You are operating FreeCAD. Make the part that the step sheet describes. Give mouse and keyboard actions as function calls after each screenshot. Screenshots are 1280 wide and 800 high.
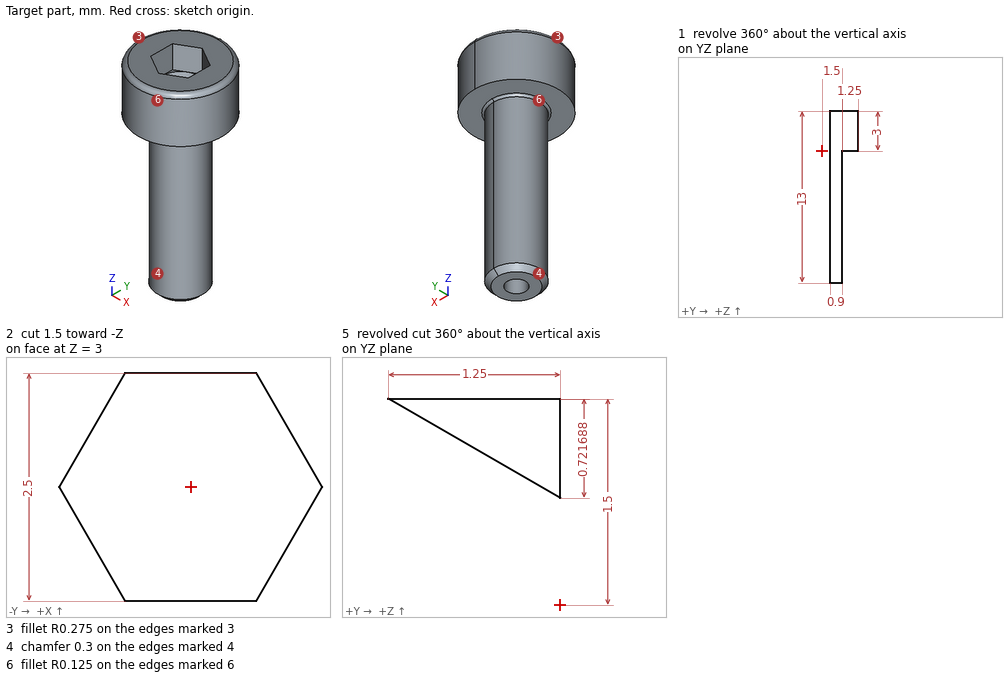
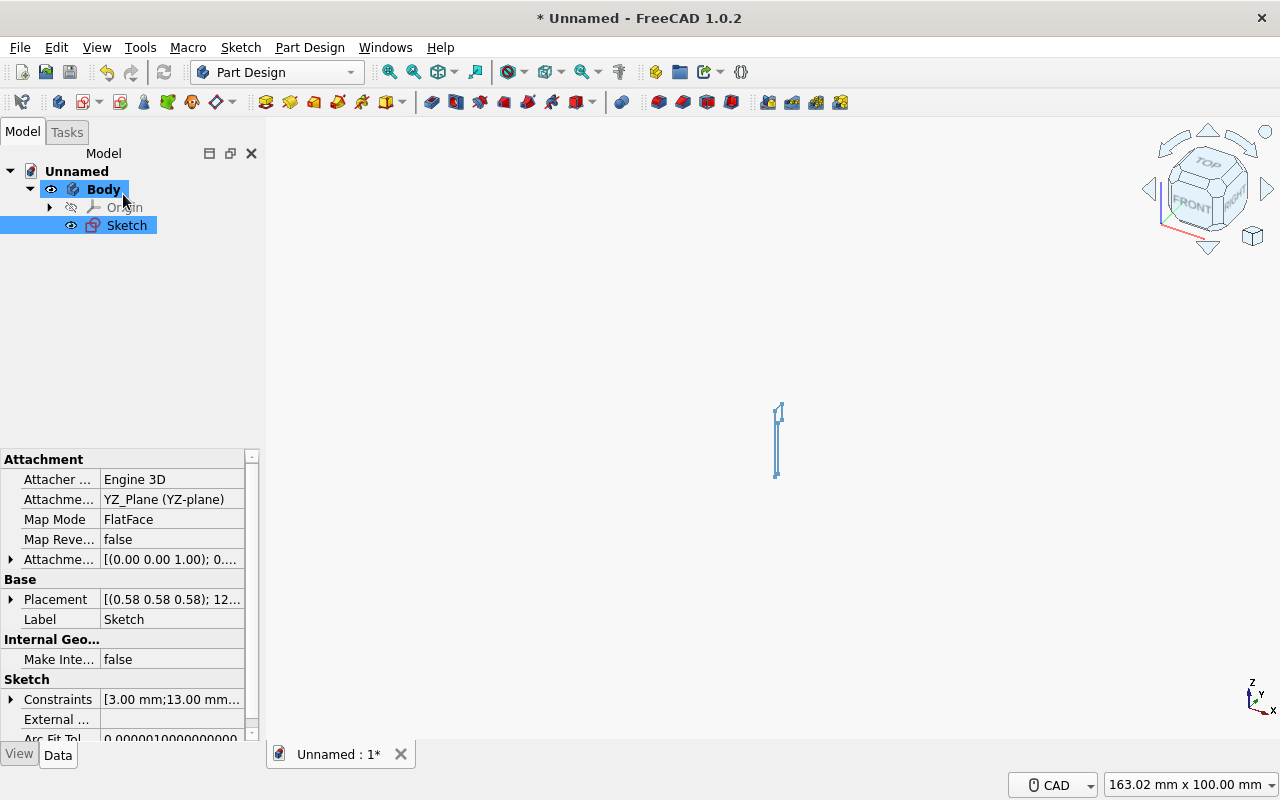
click(290, 102)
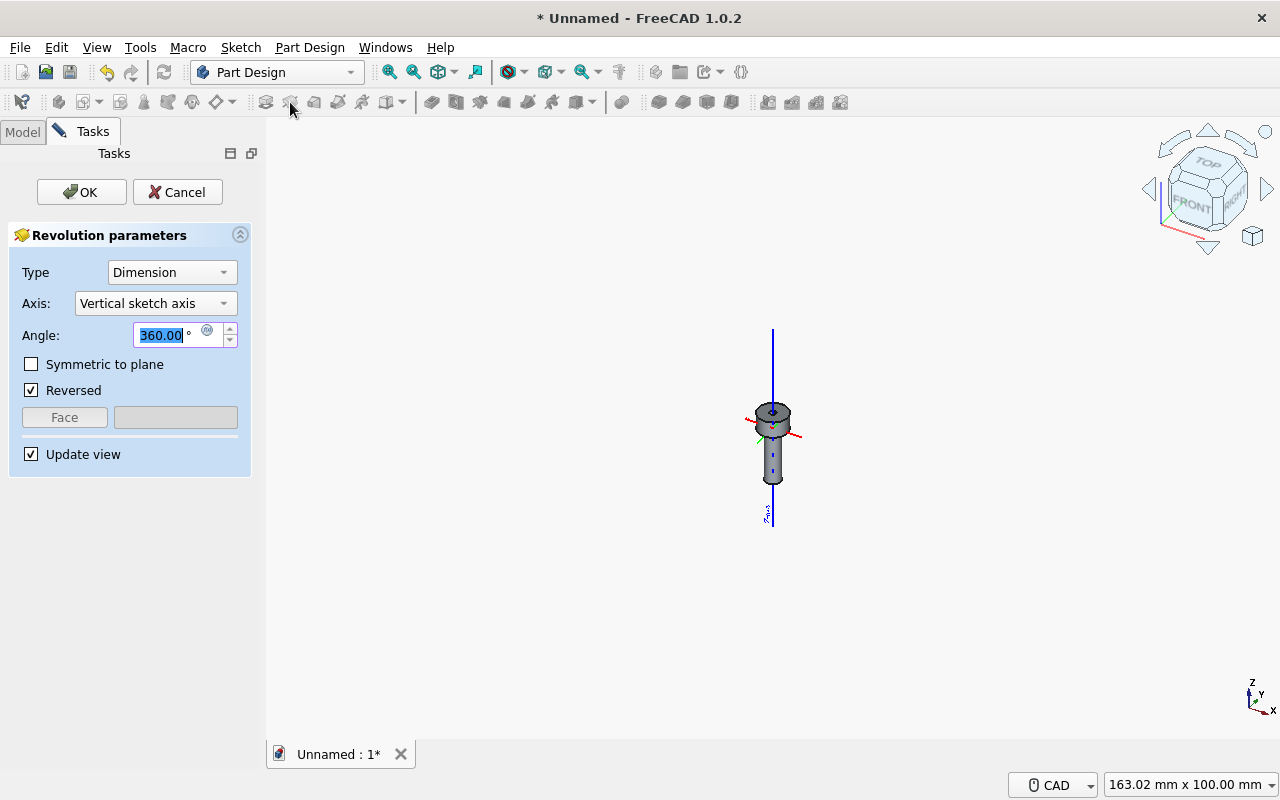
click(82, 192)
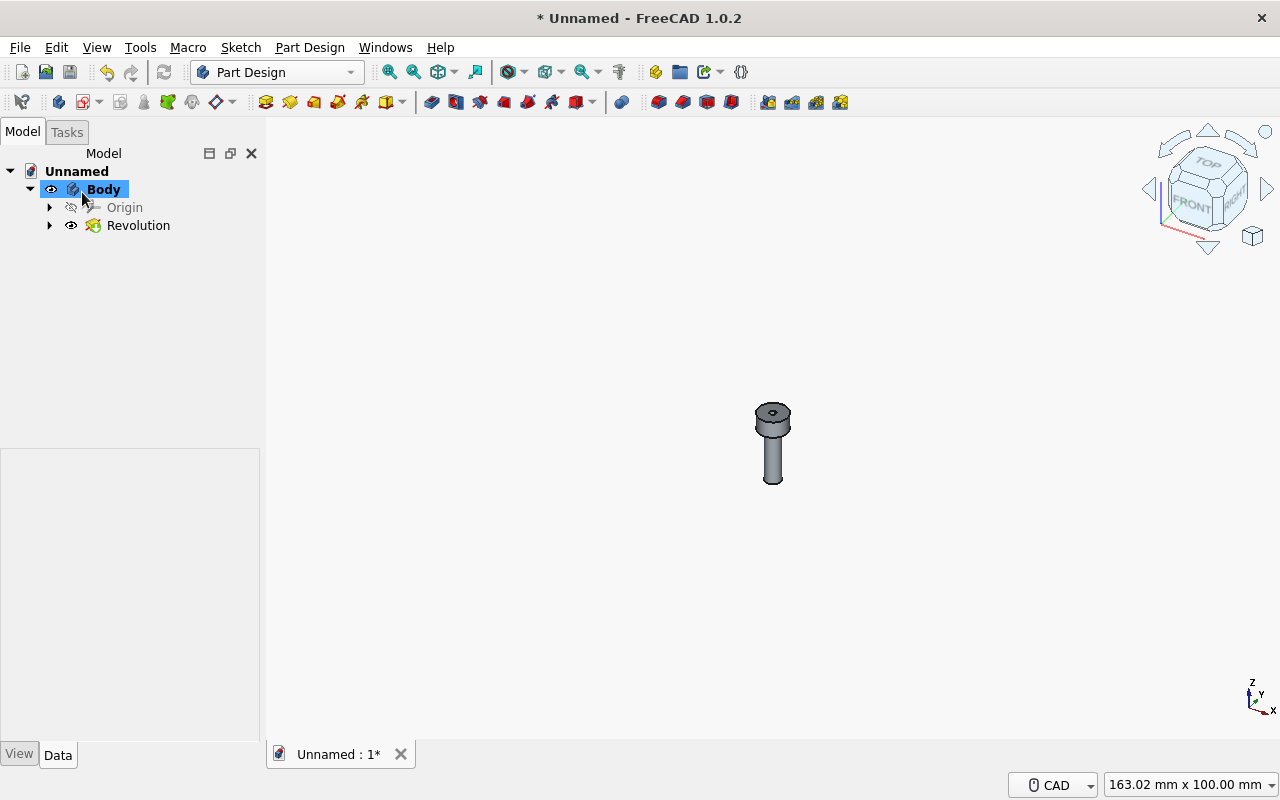
click(390, 72)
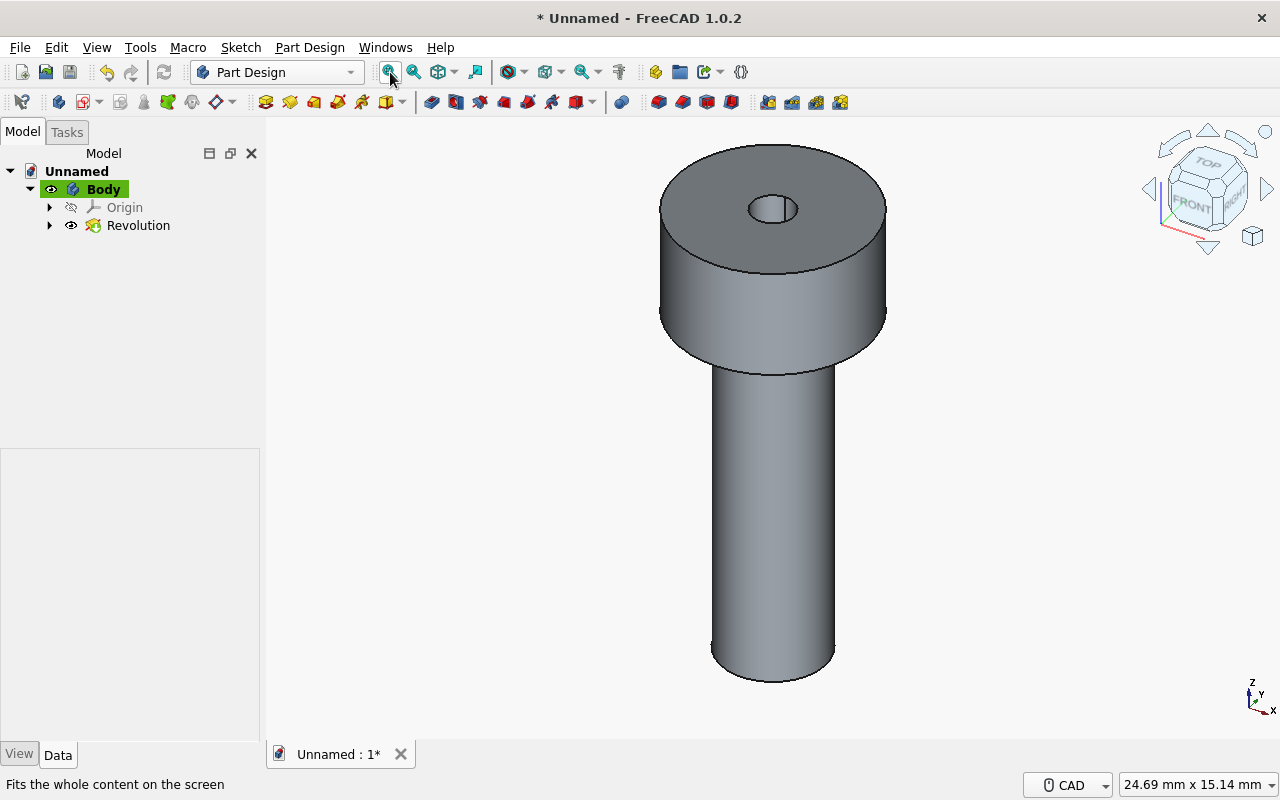
click(845, 211)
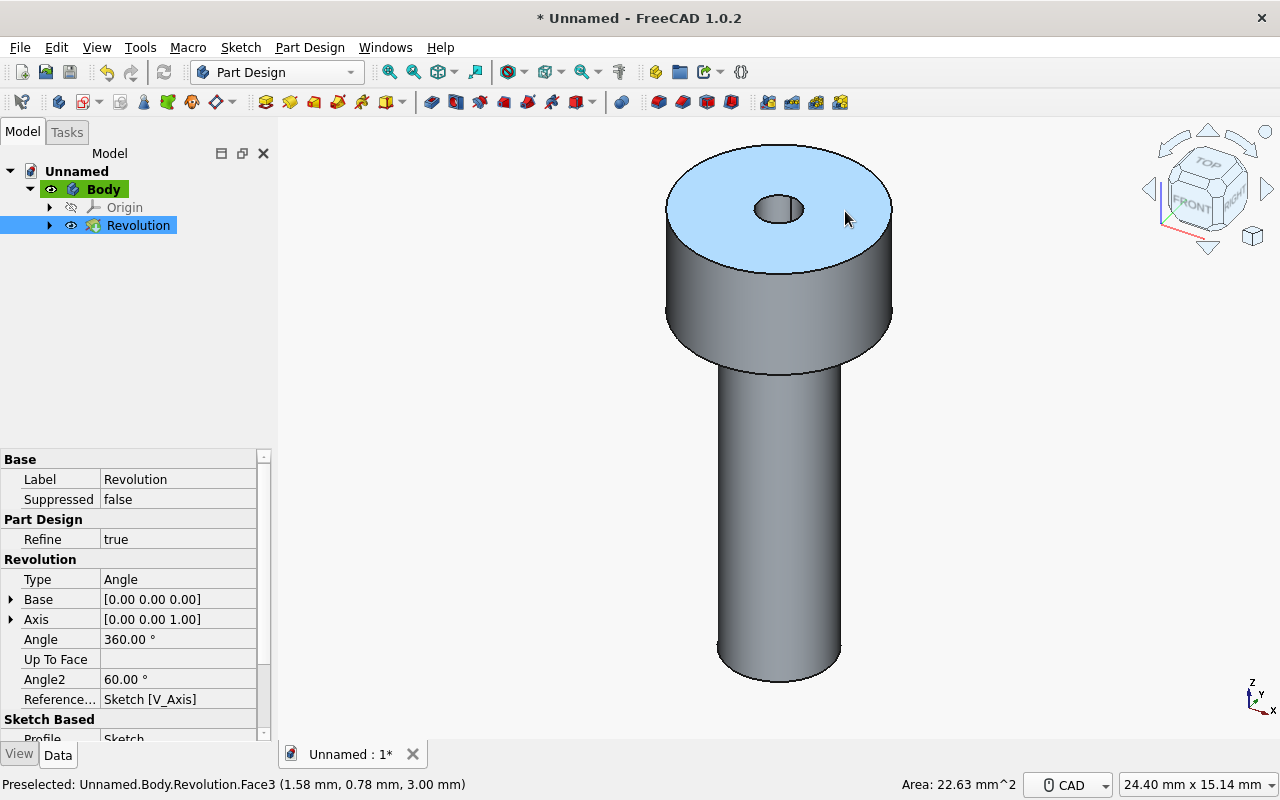
click(84, 102)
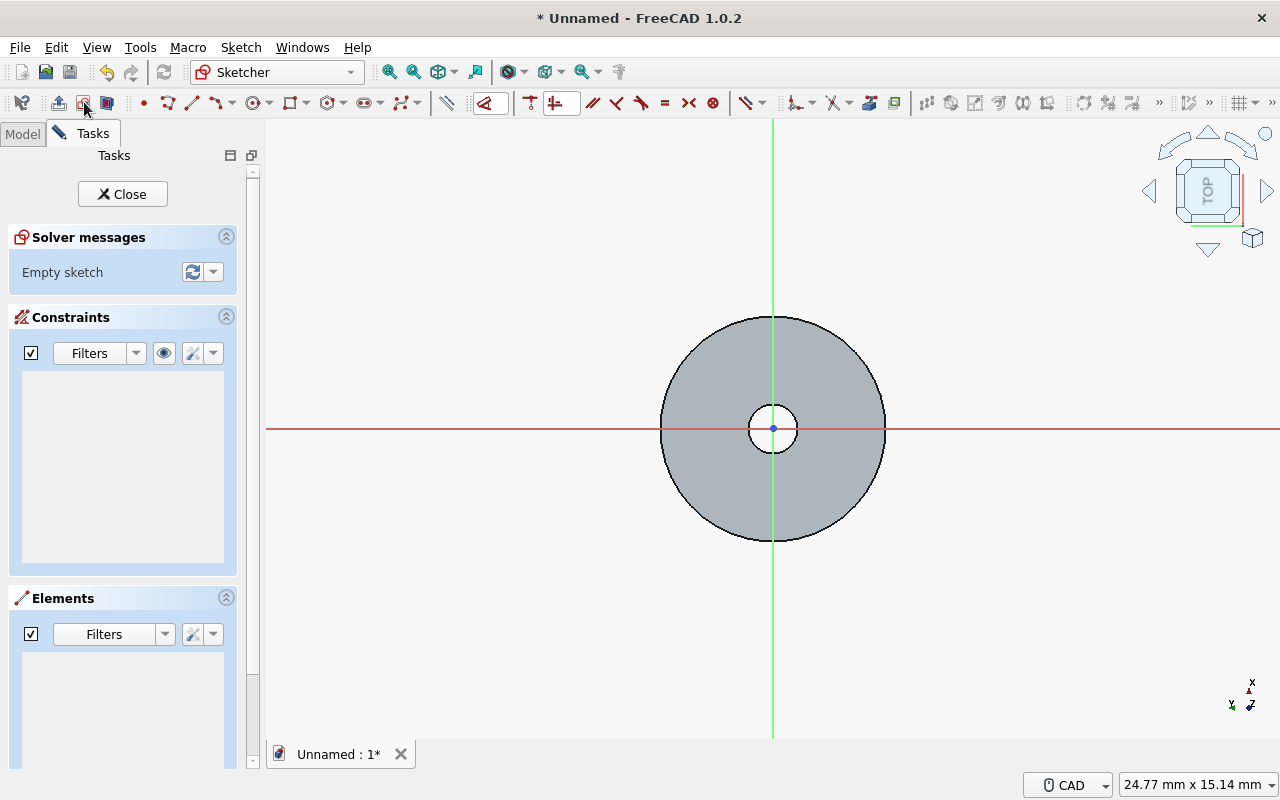
scroll(795, 429, up, 7)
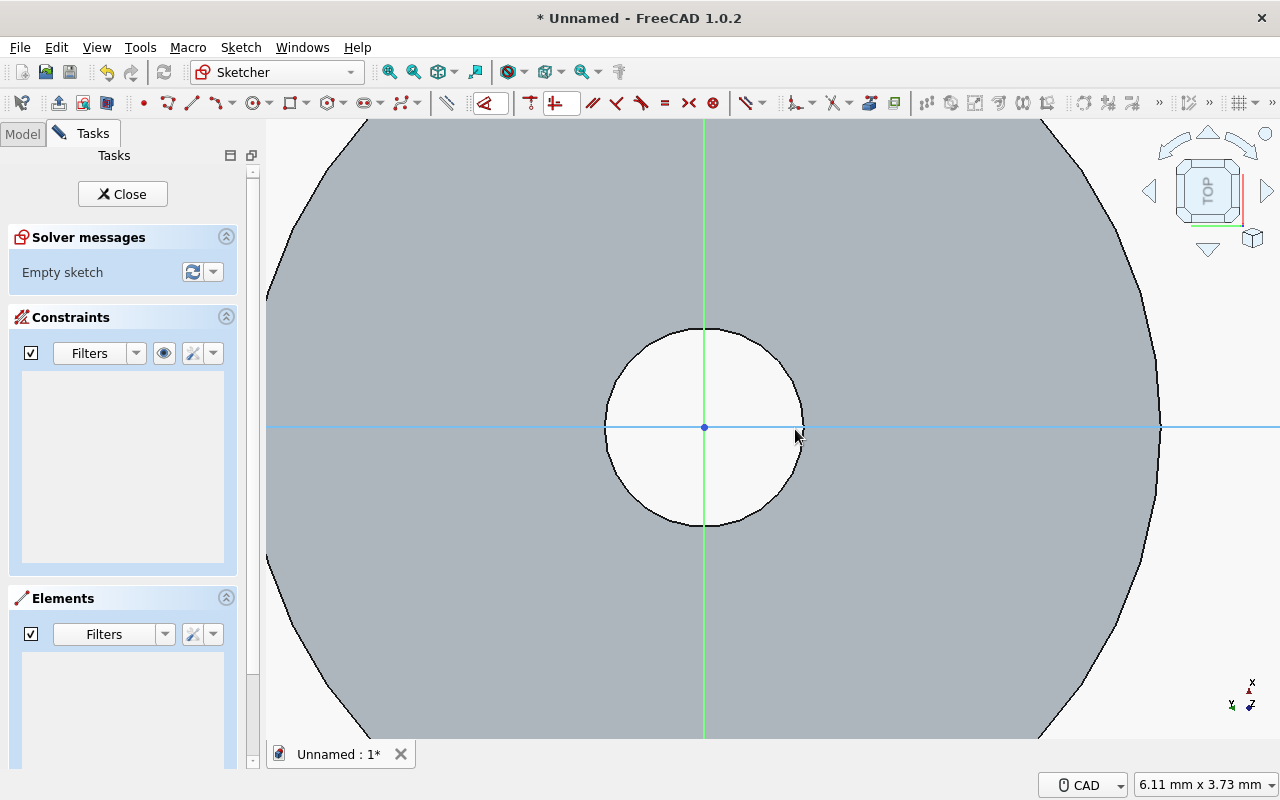
click(328, 104)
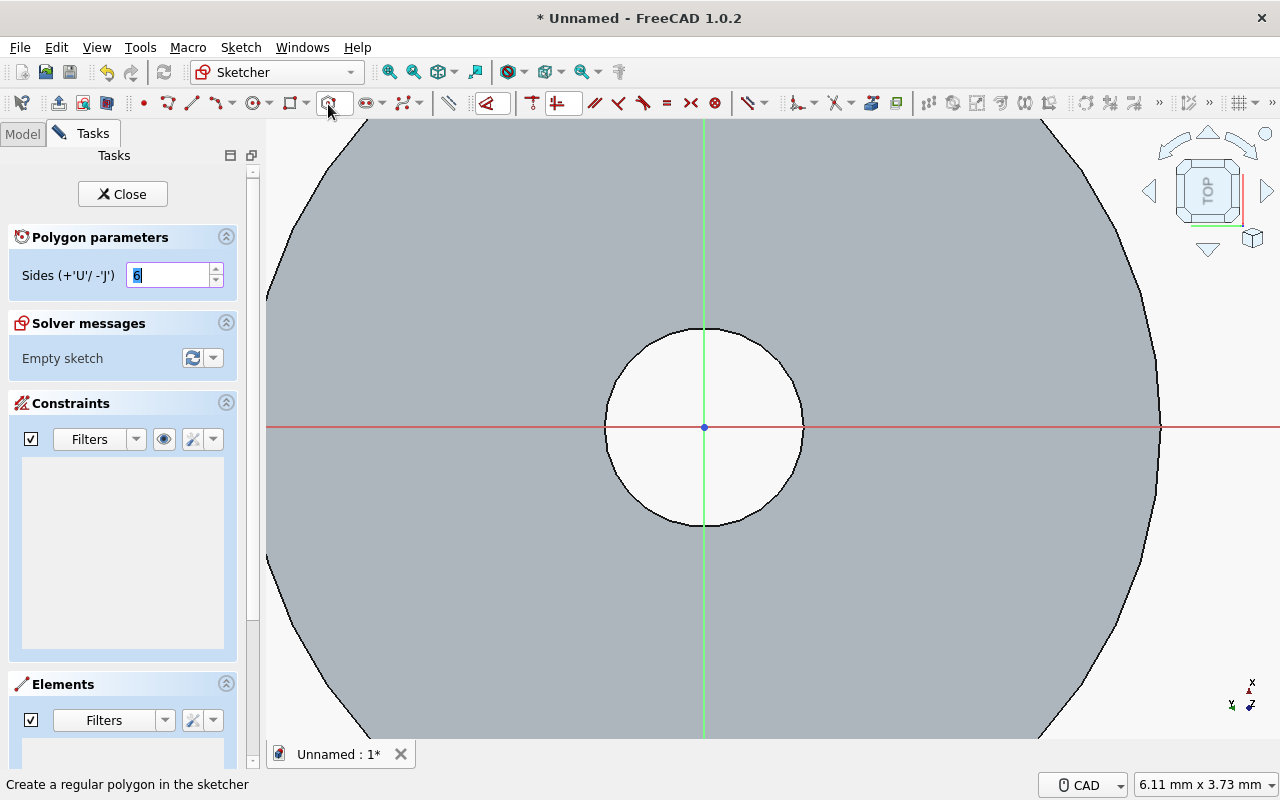
click(704, 427)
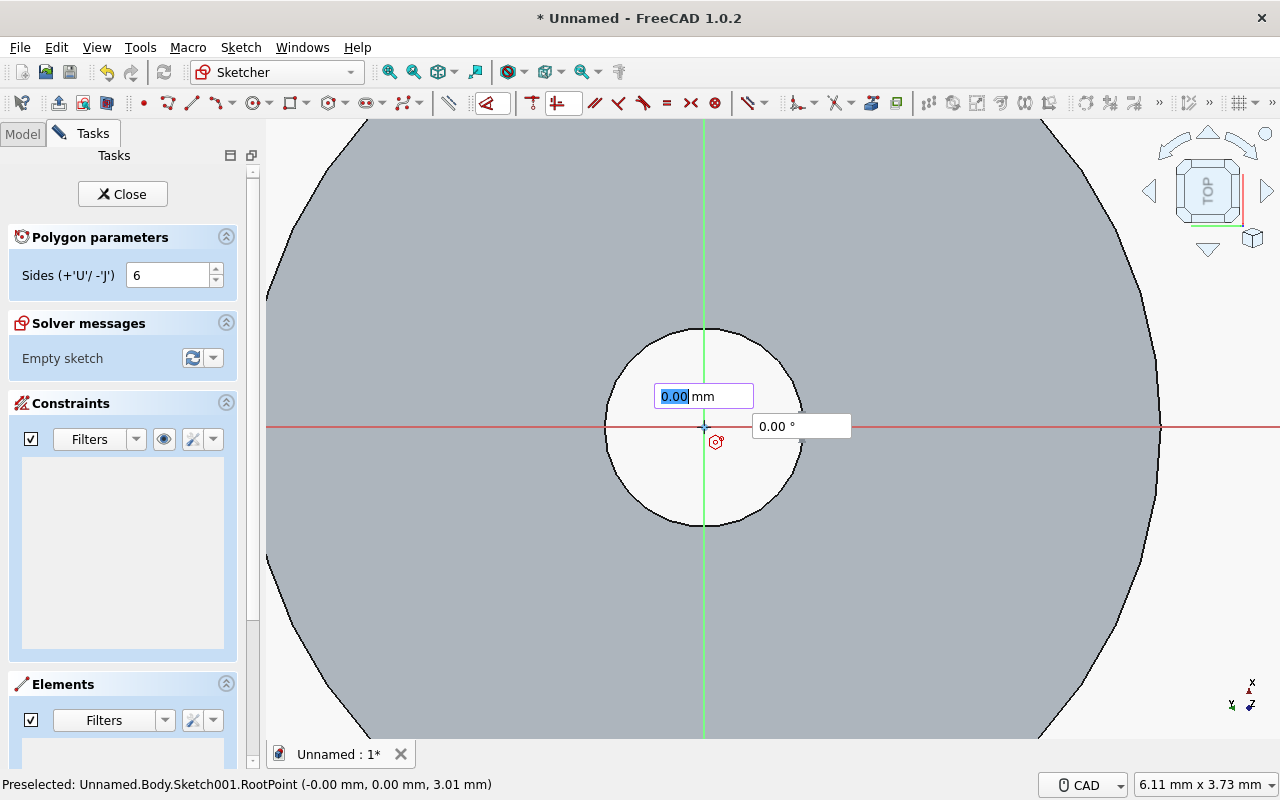
click(465, 427)
key(Escape)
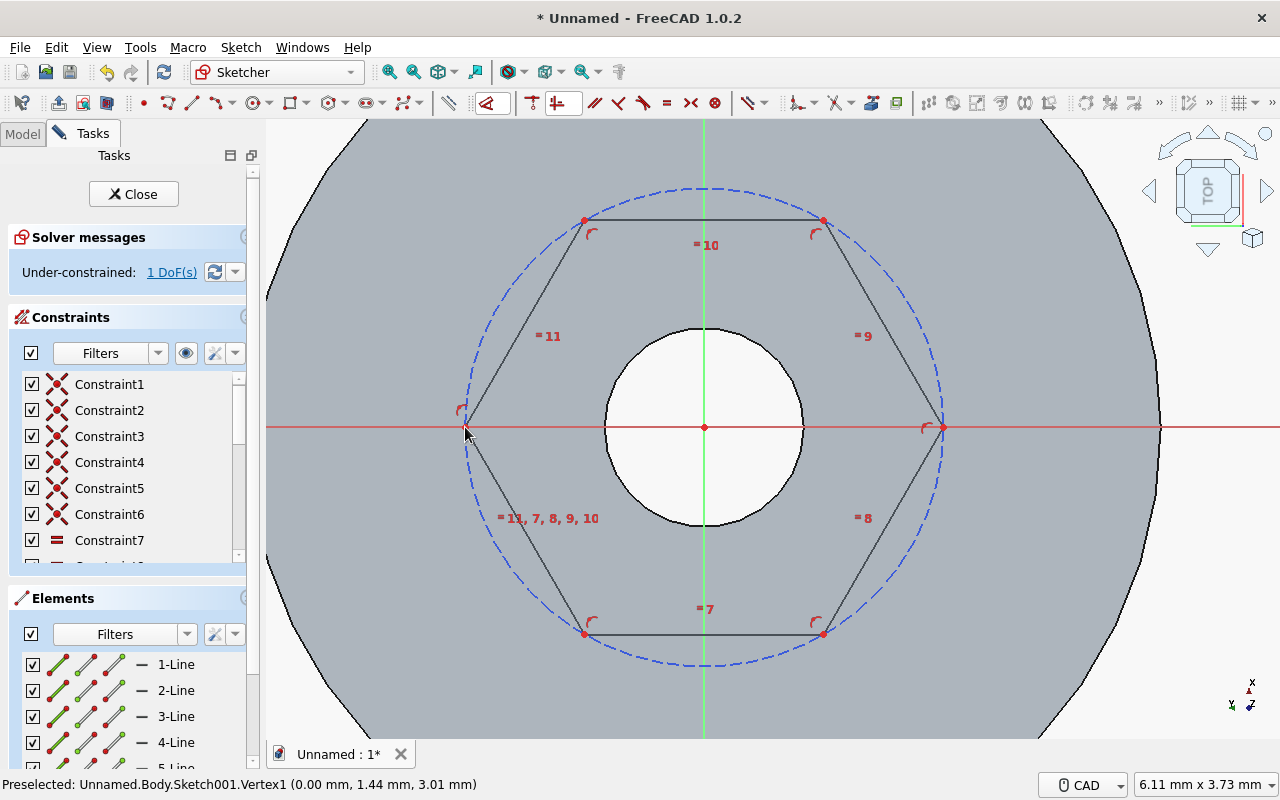
click(585, 635)